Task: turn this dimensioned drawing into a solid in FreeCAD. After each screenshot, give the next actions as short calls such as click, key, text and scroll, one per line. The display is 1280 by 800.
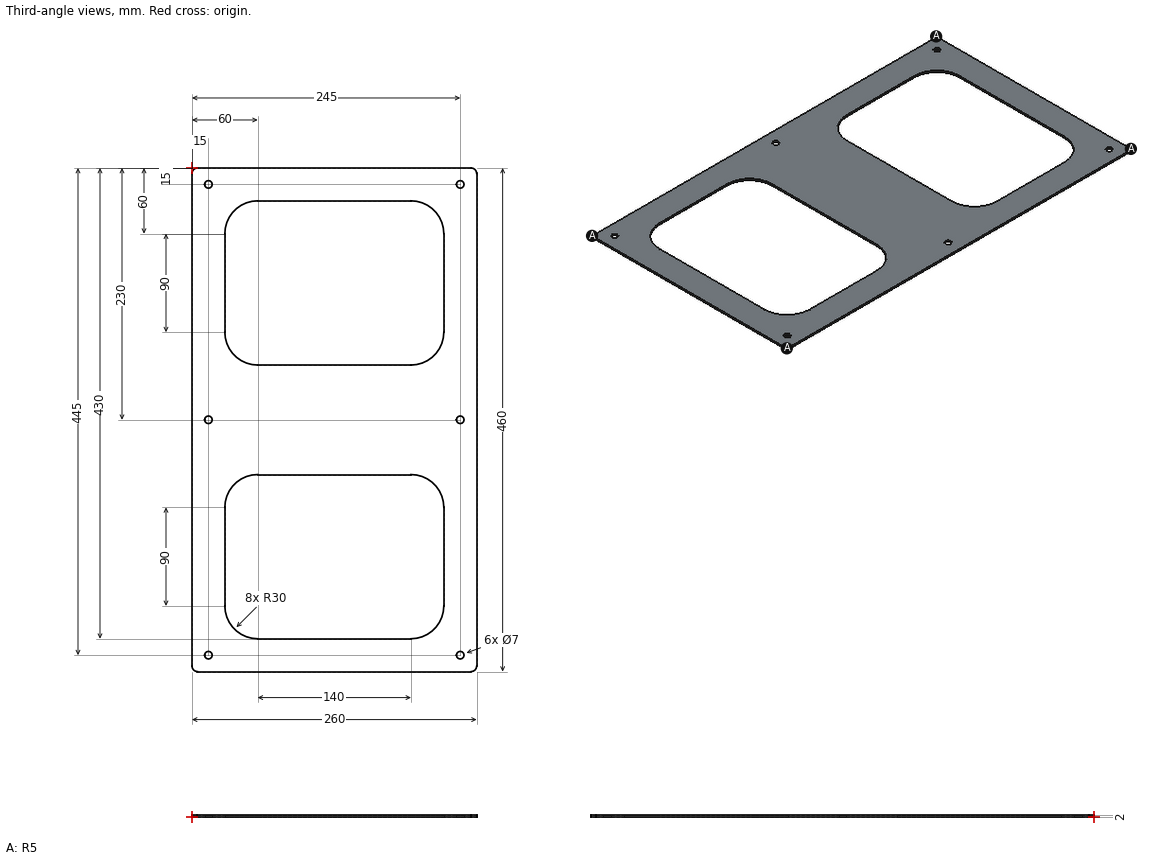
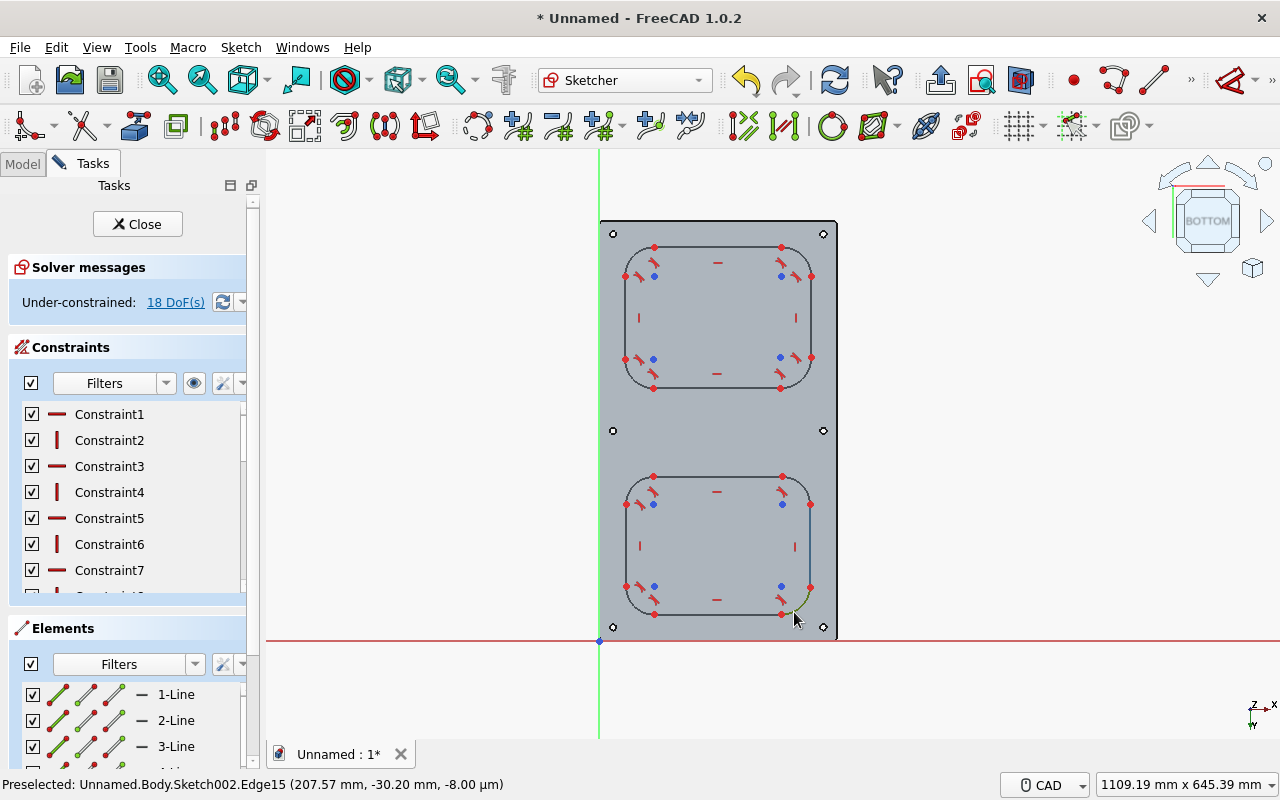
key(t)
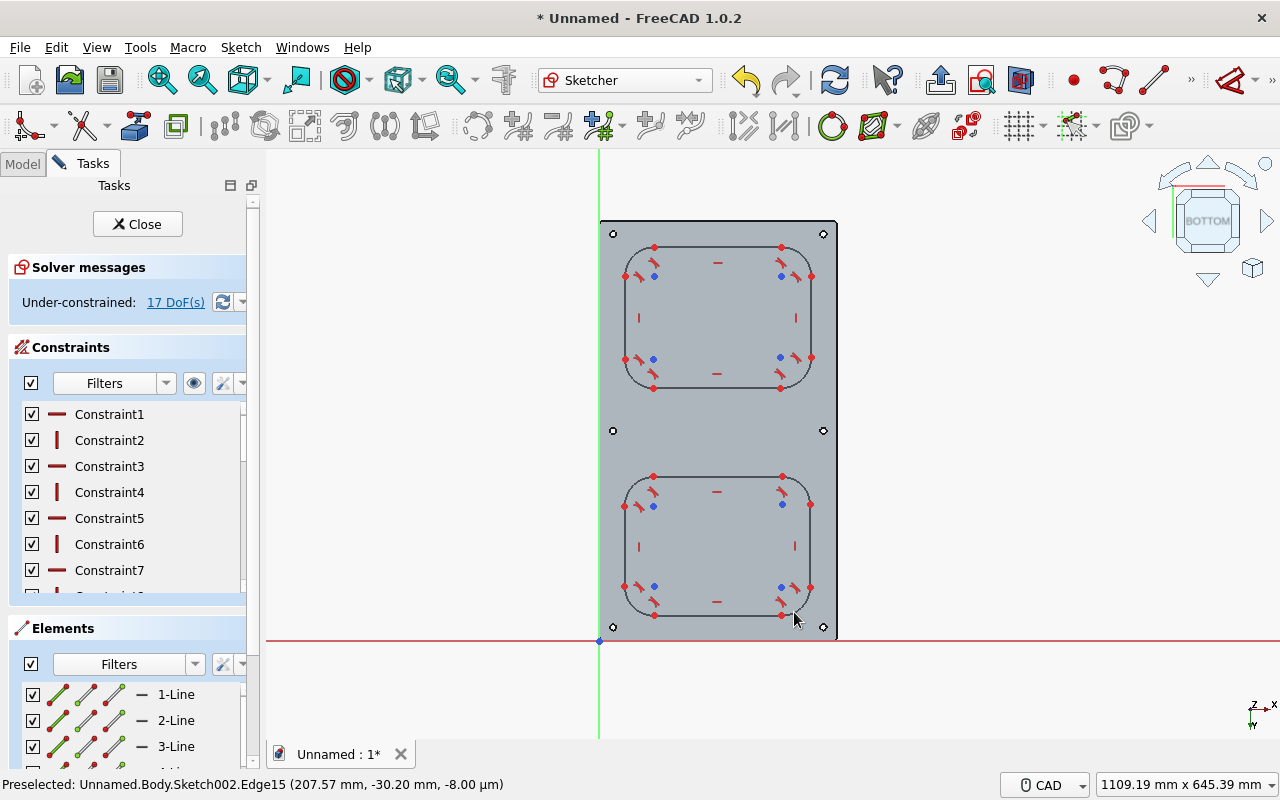
click(810, 562)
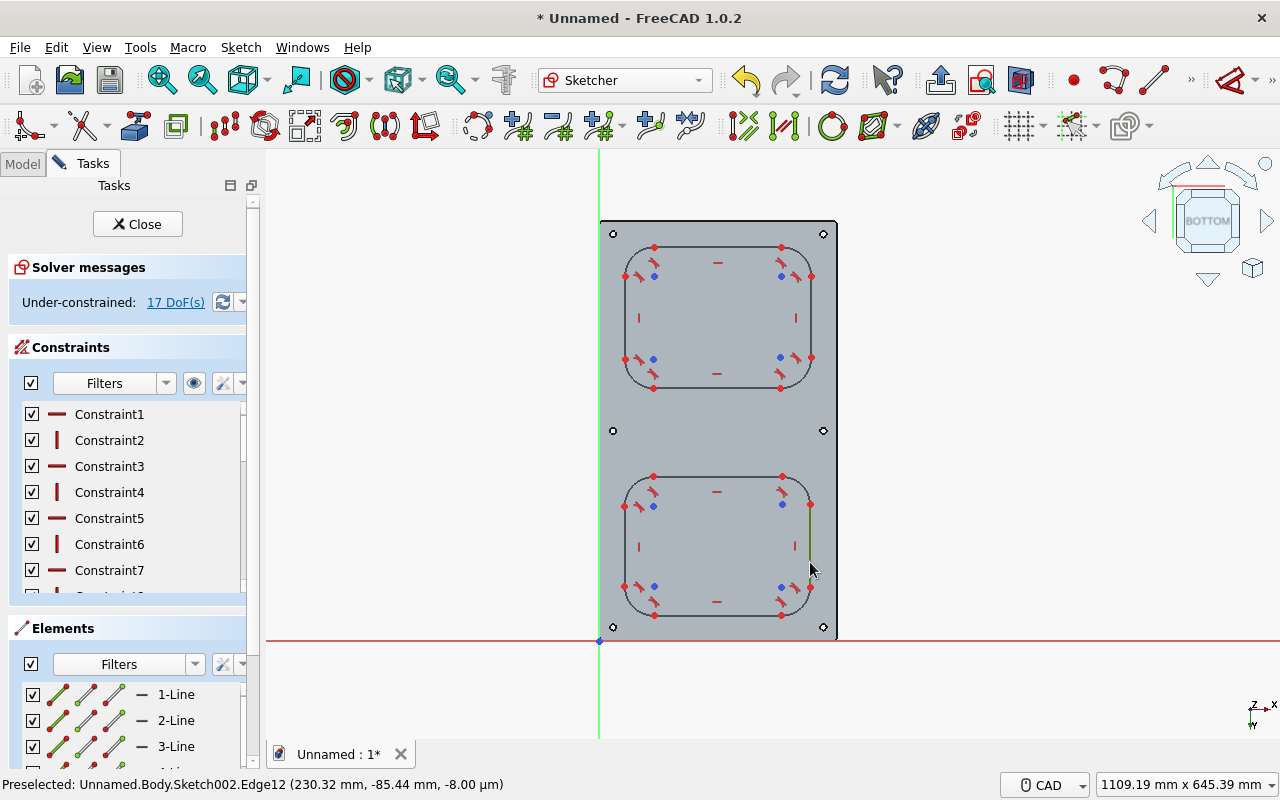
click(807, 492)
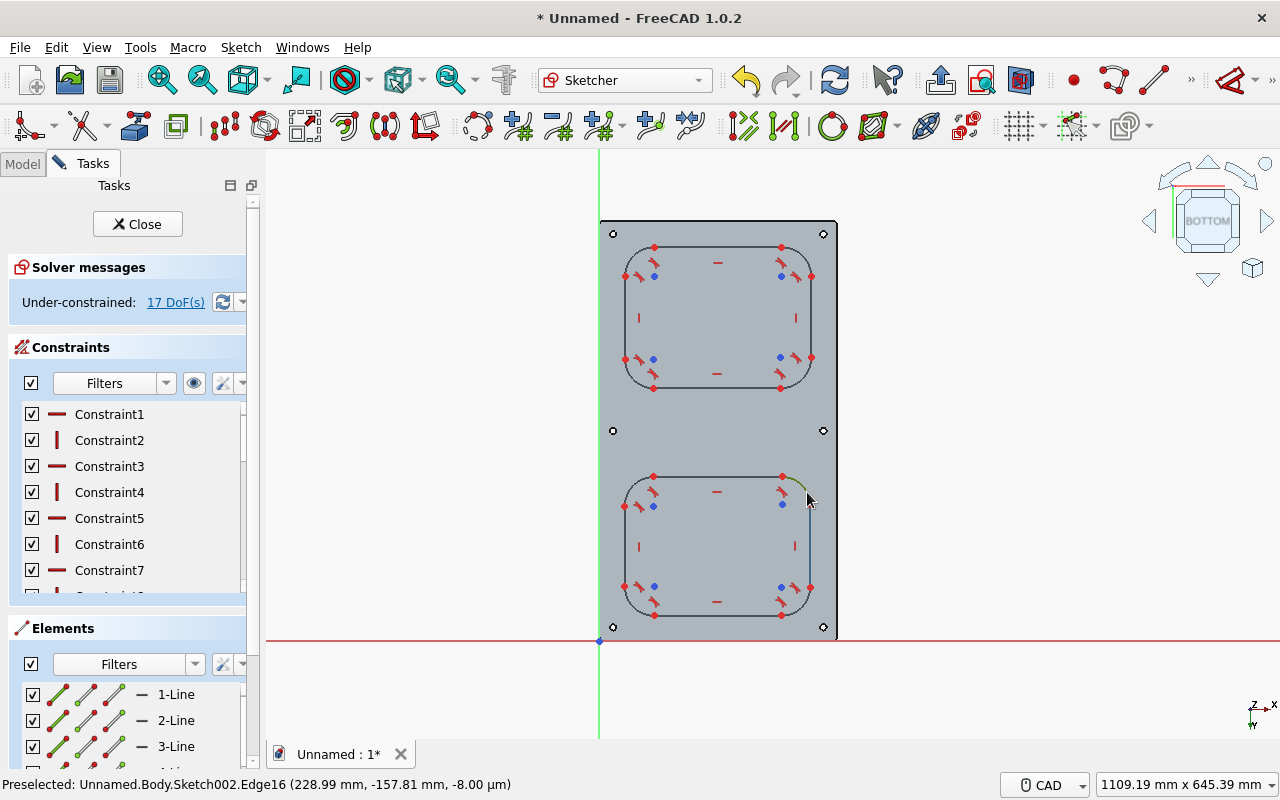
key(t)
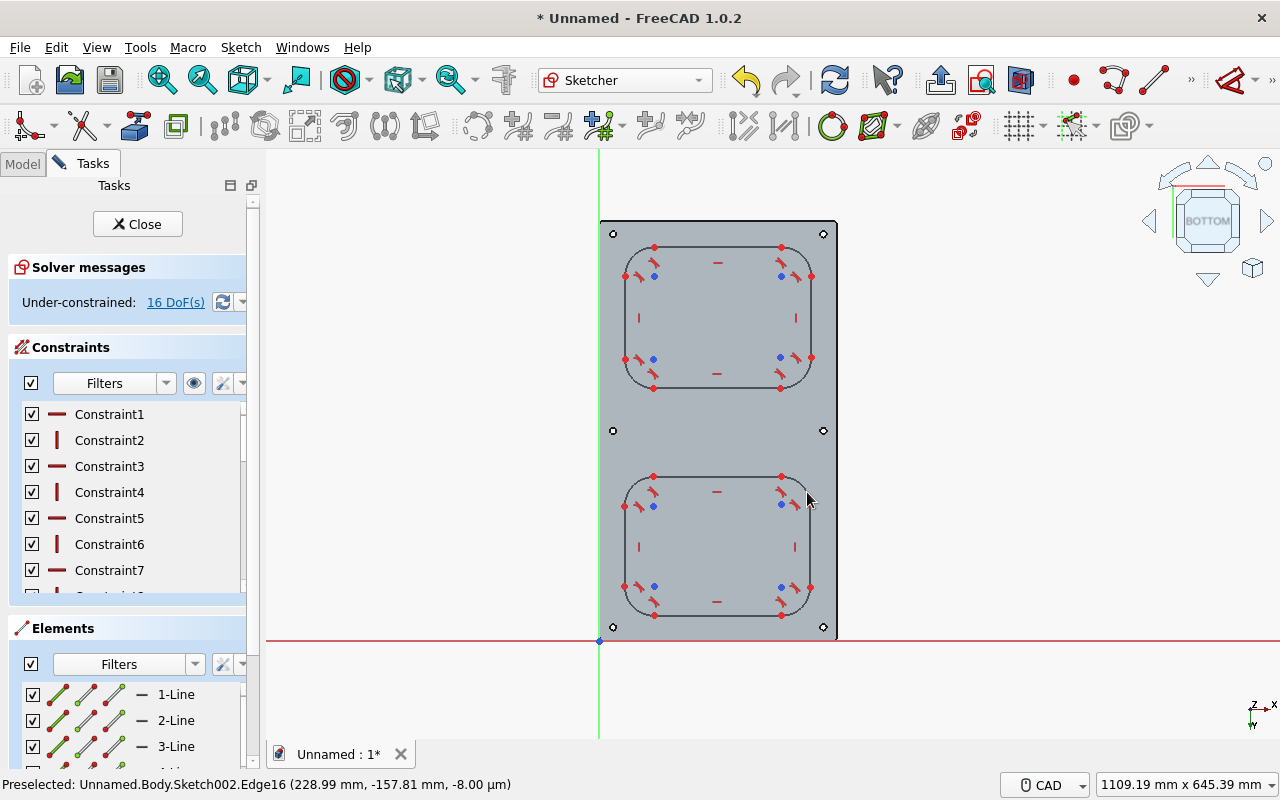
click(641, 250)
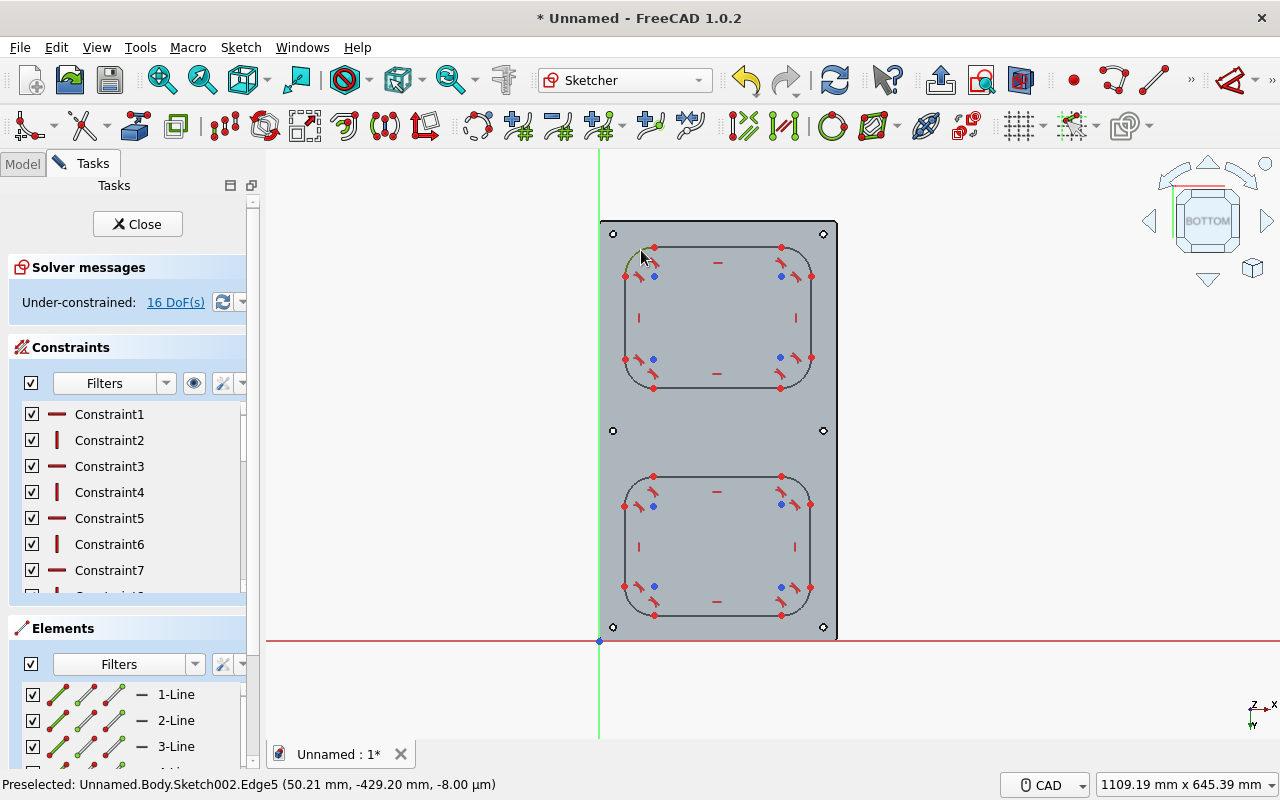
click(628, 372)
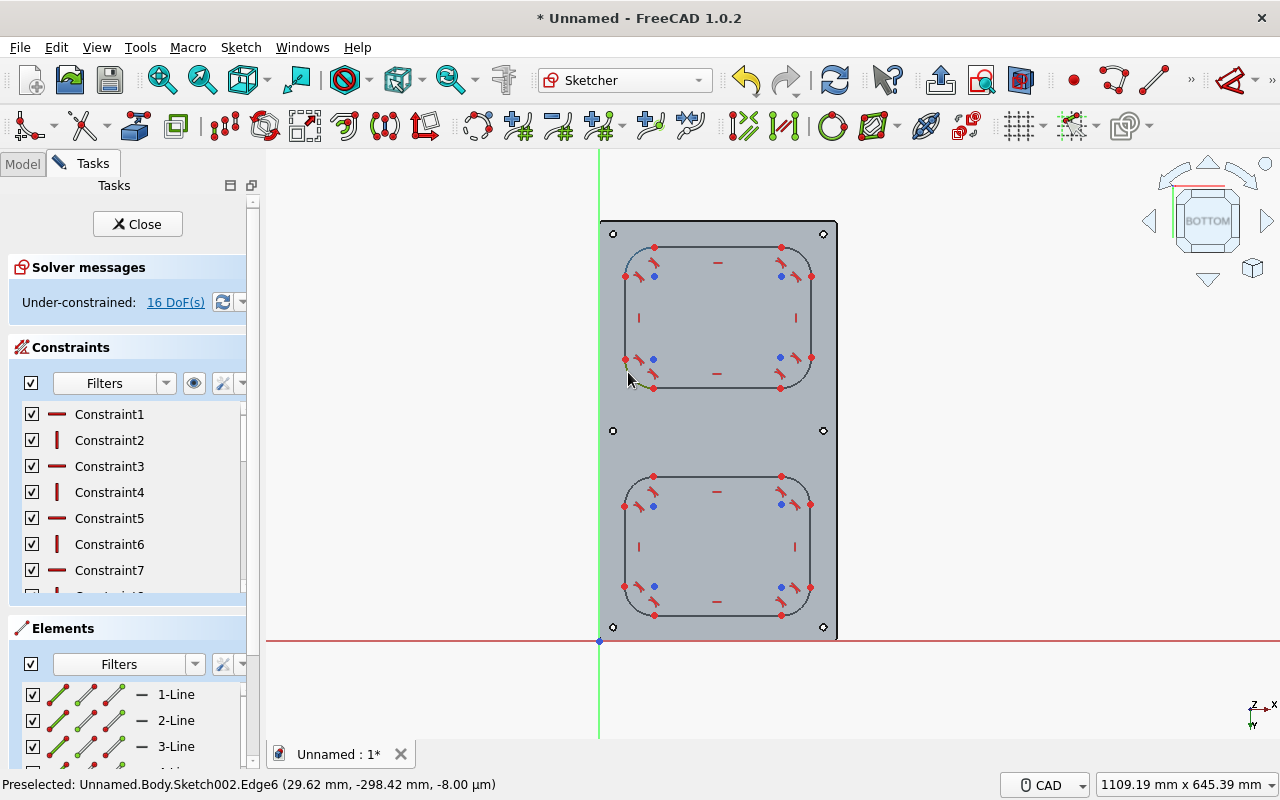
click(794, 385)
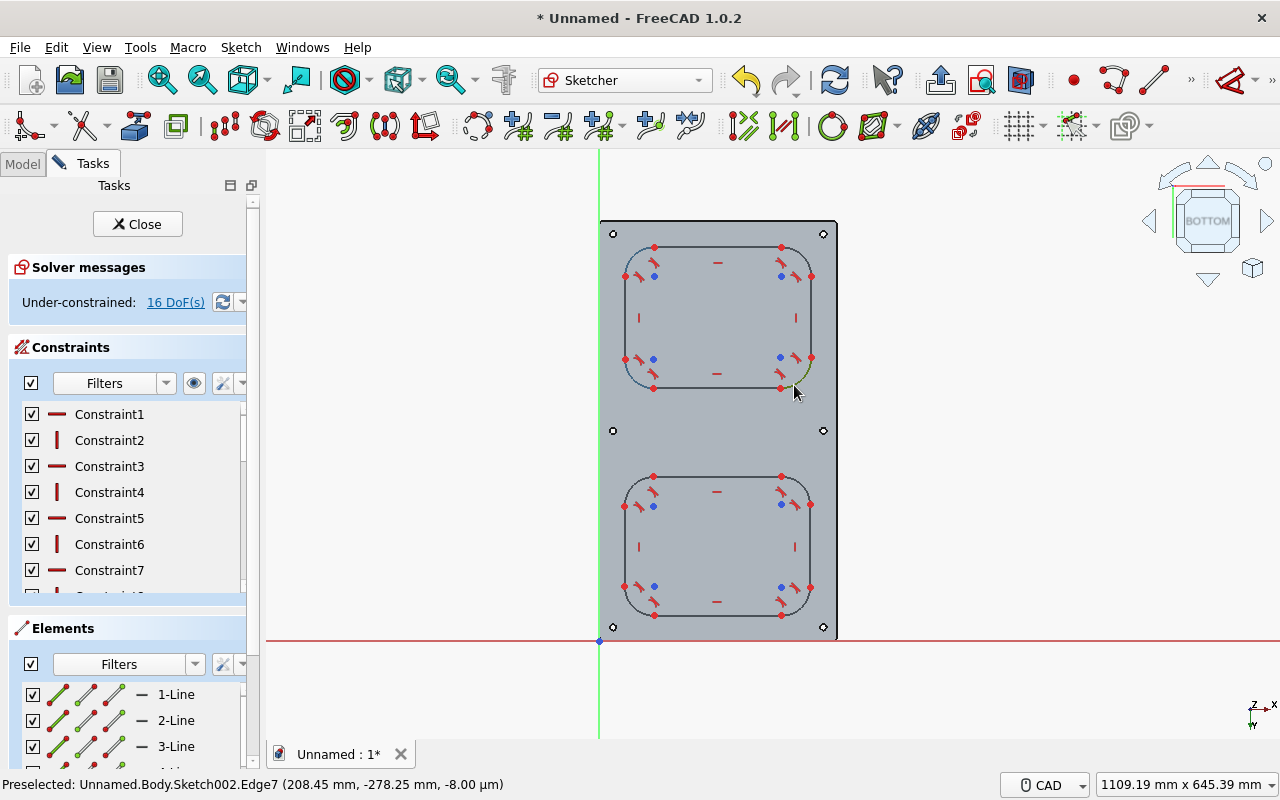
click(808, 263)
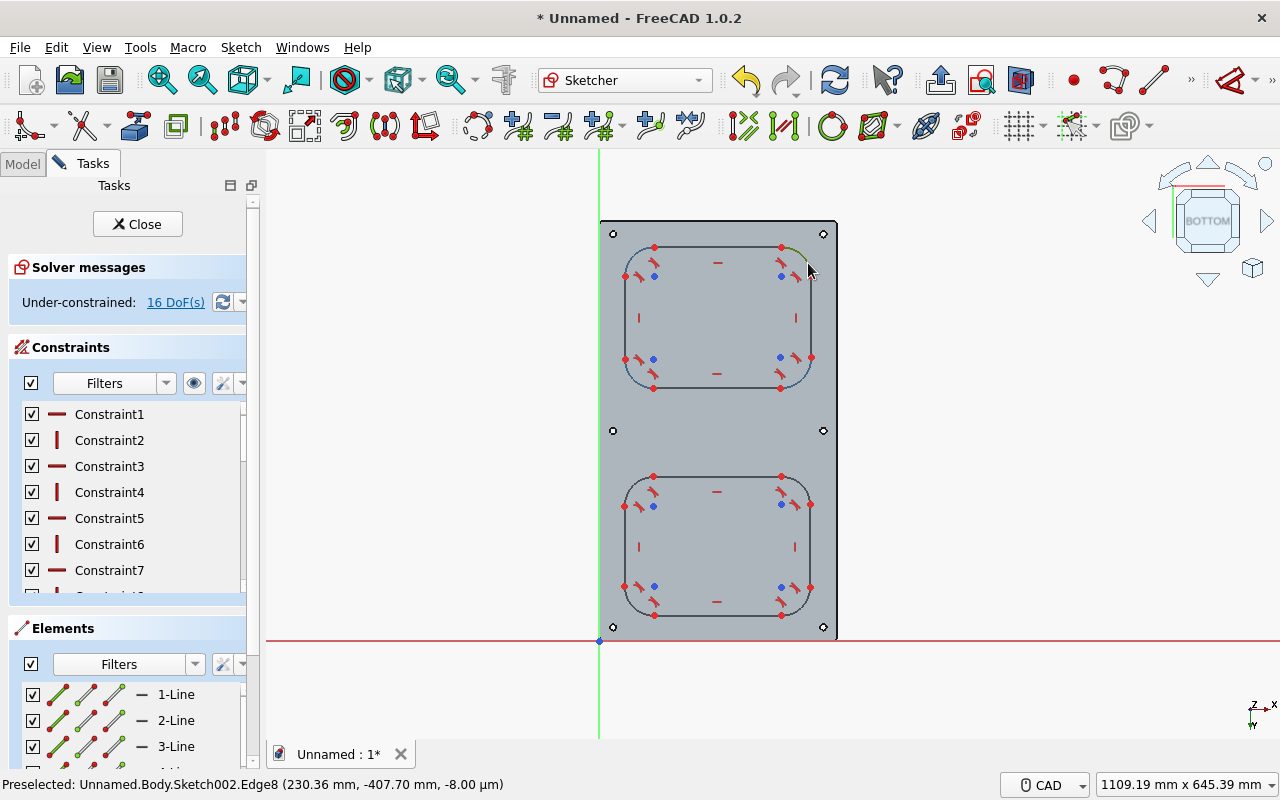
click(641, 480)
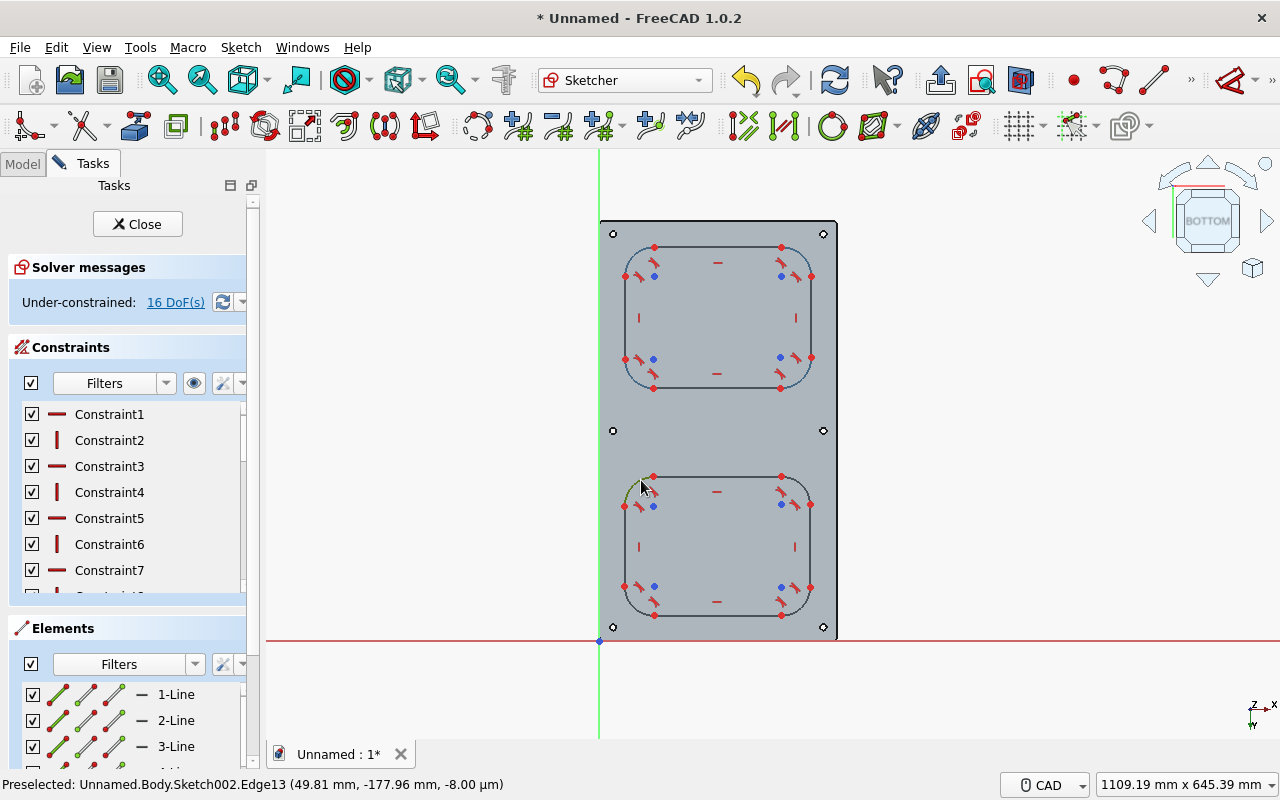
click(628, 600)